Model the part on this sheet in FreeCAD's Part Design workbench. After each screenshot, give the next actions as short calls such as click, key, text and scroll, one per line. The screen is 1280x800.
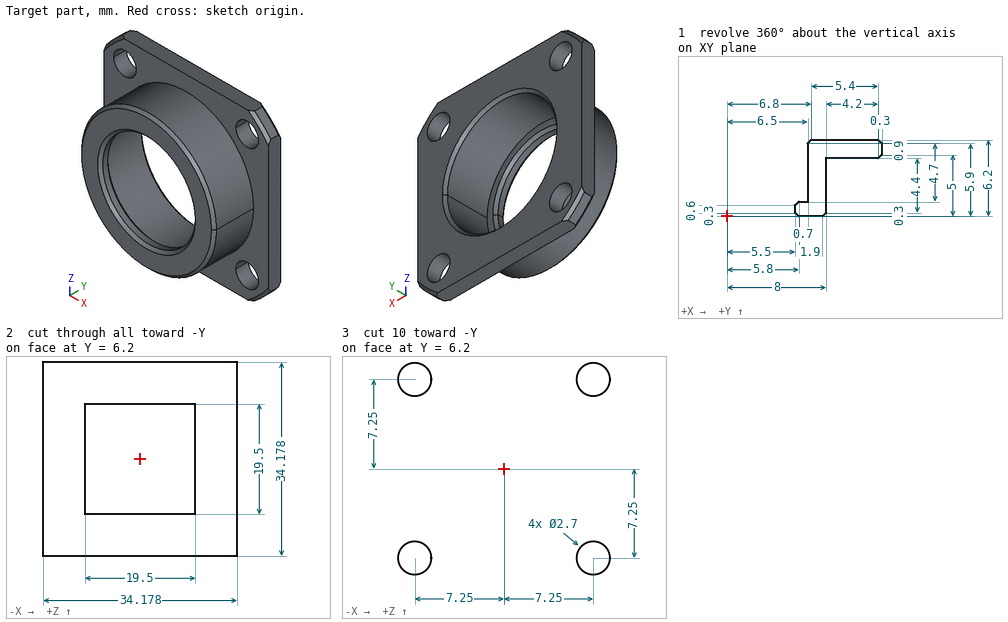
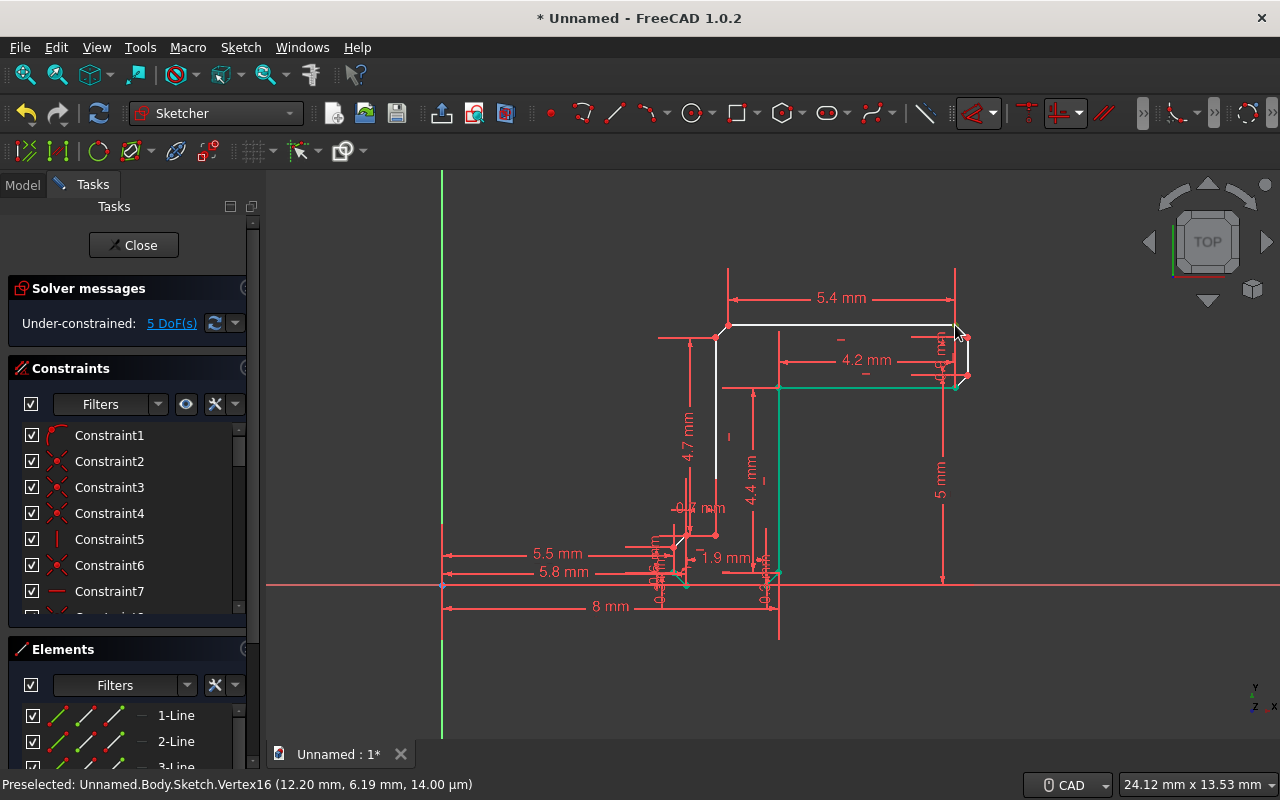
click(996, 114)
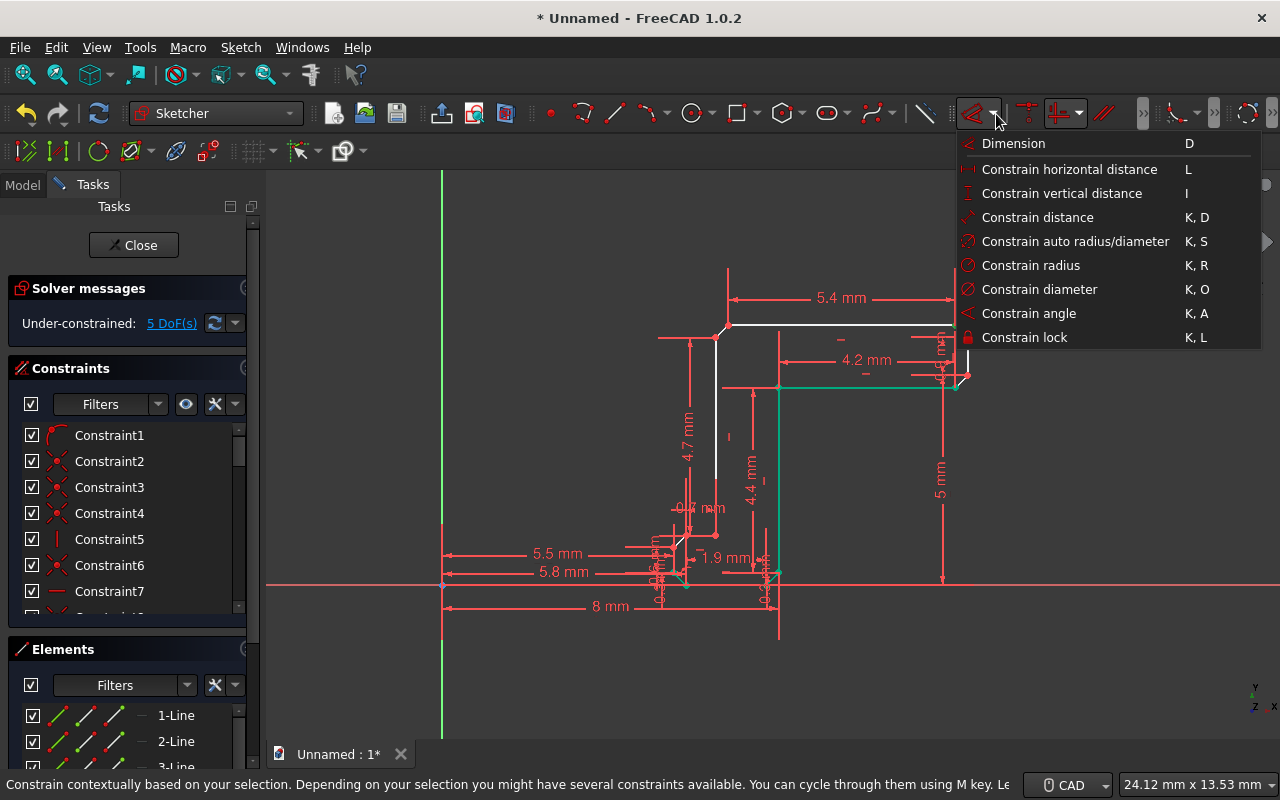
click(1109, 193)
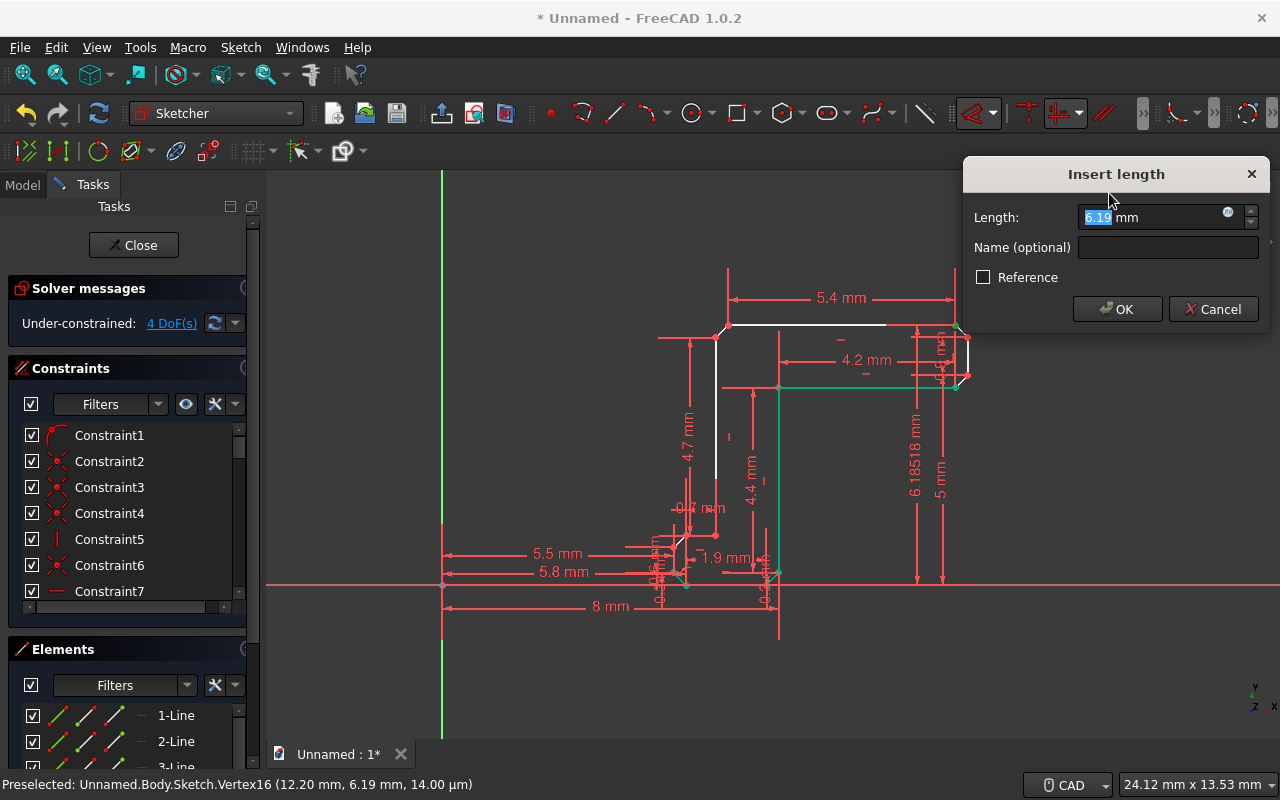
text(6.2)
key(Return)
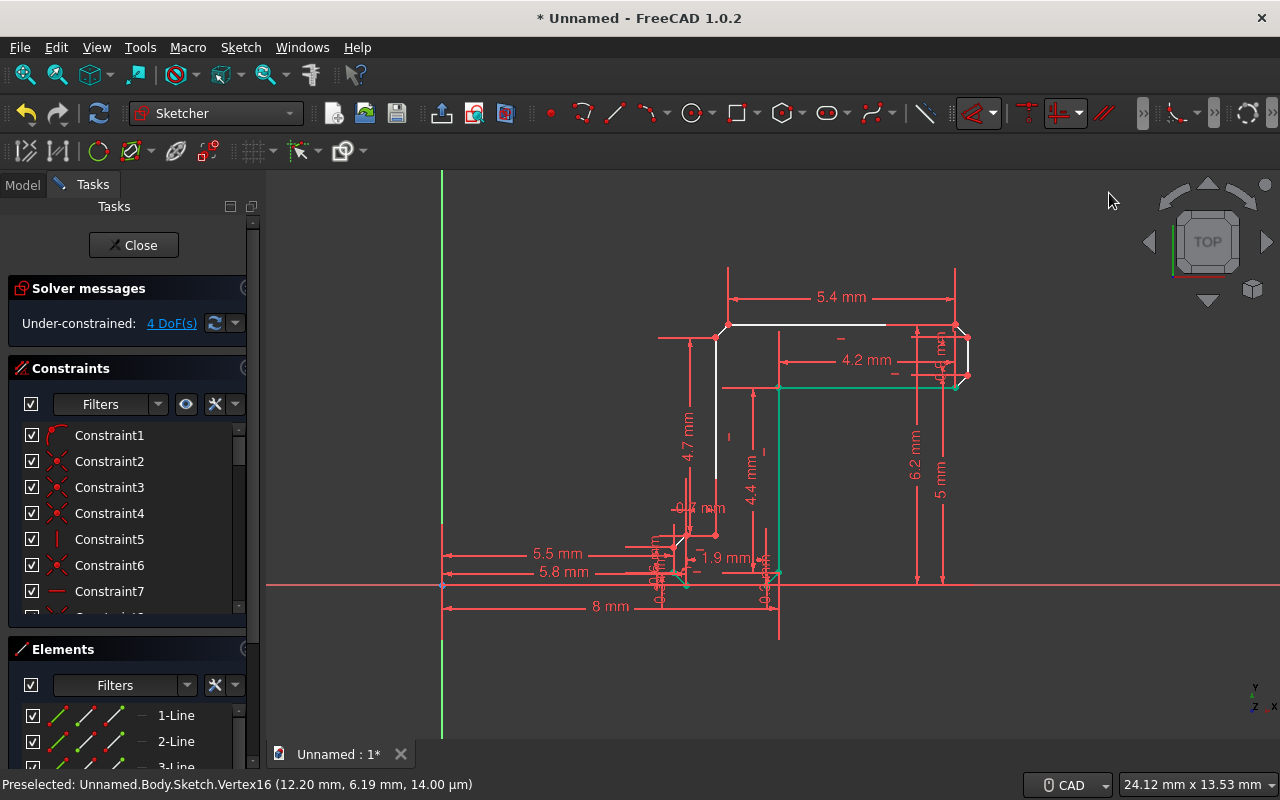
click(728, 325)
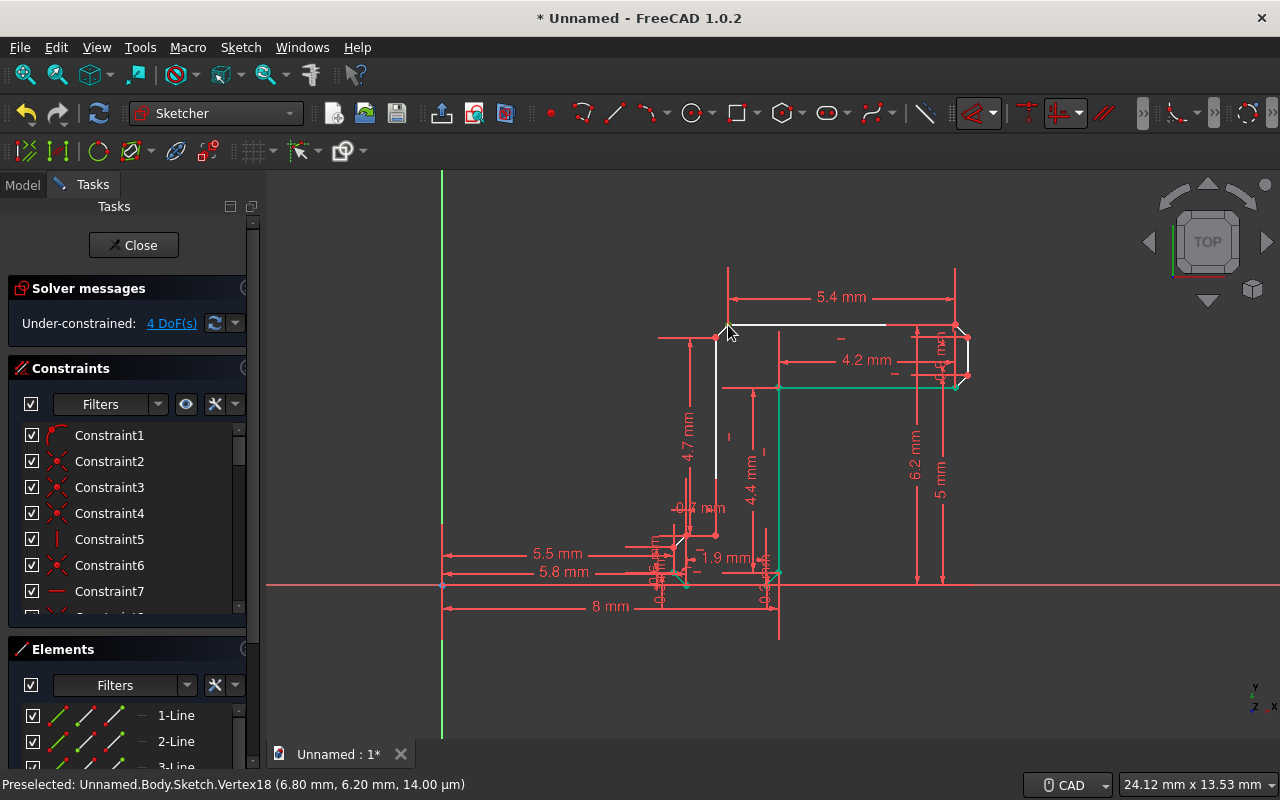
key(l)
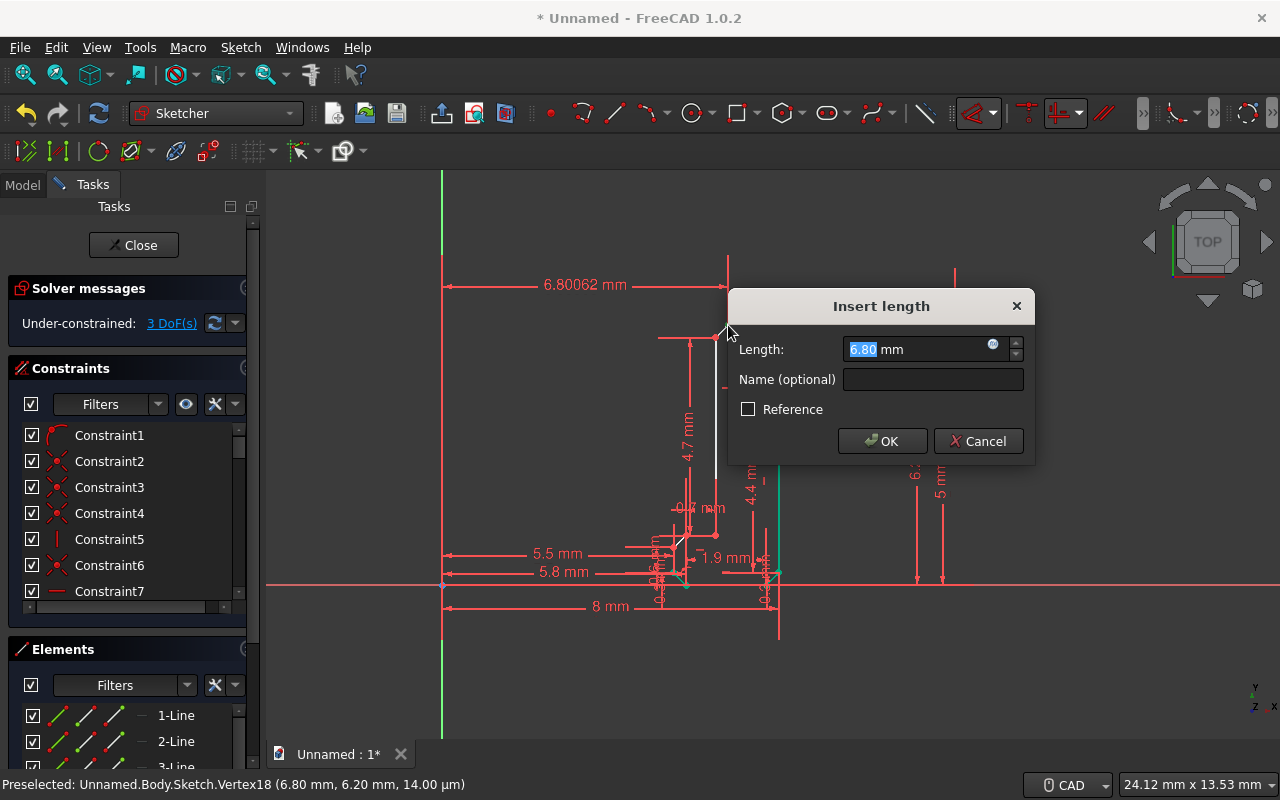
text(6.8)
key(Return)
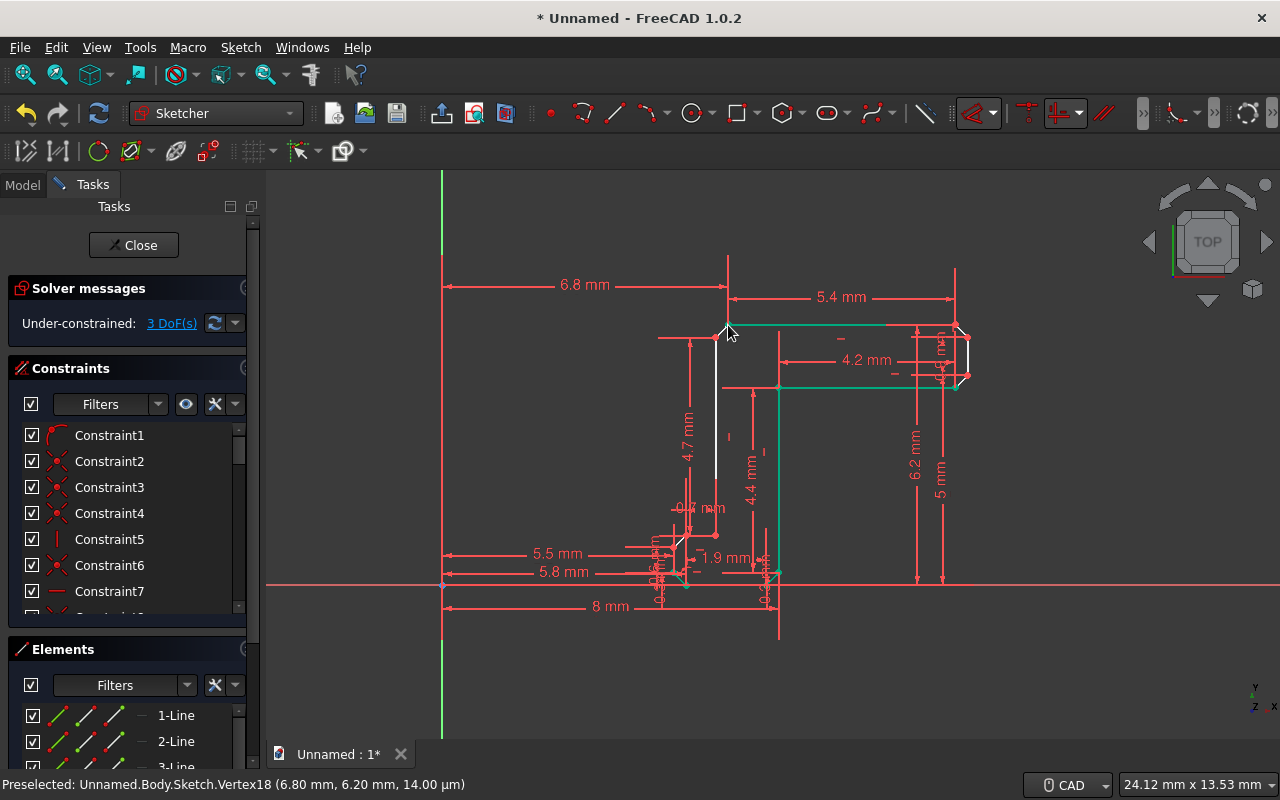
click(716, 338)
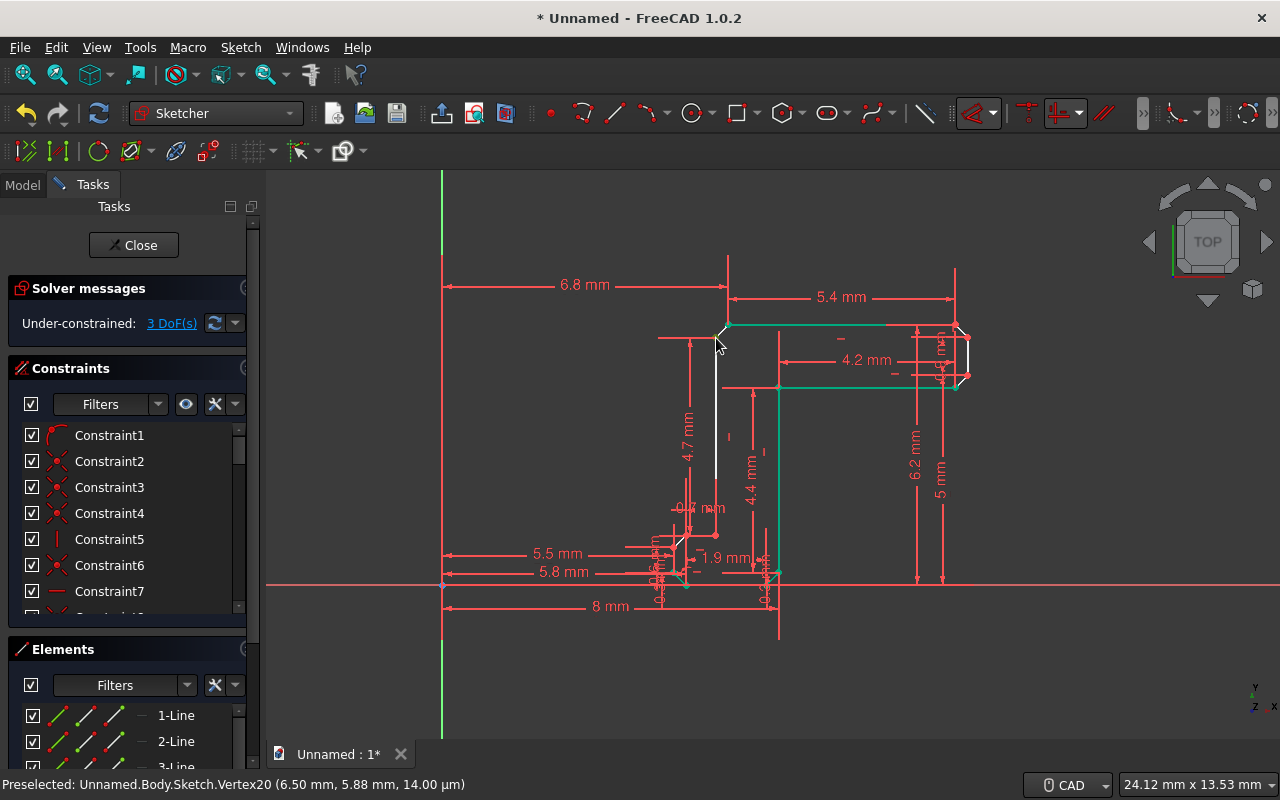
click(996, 114)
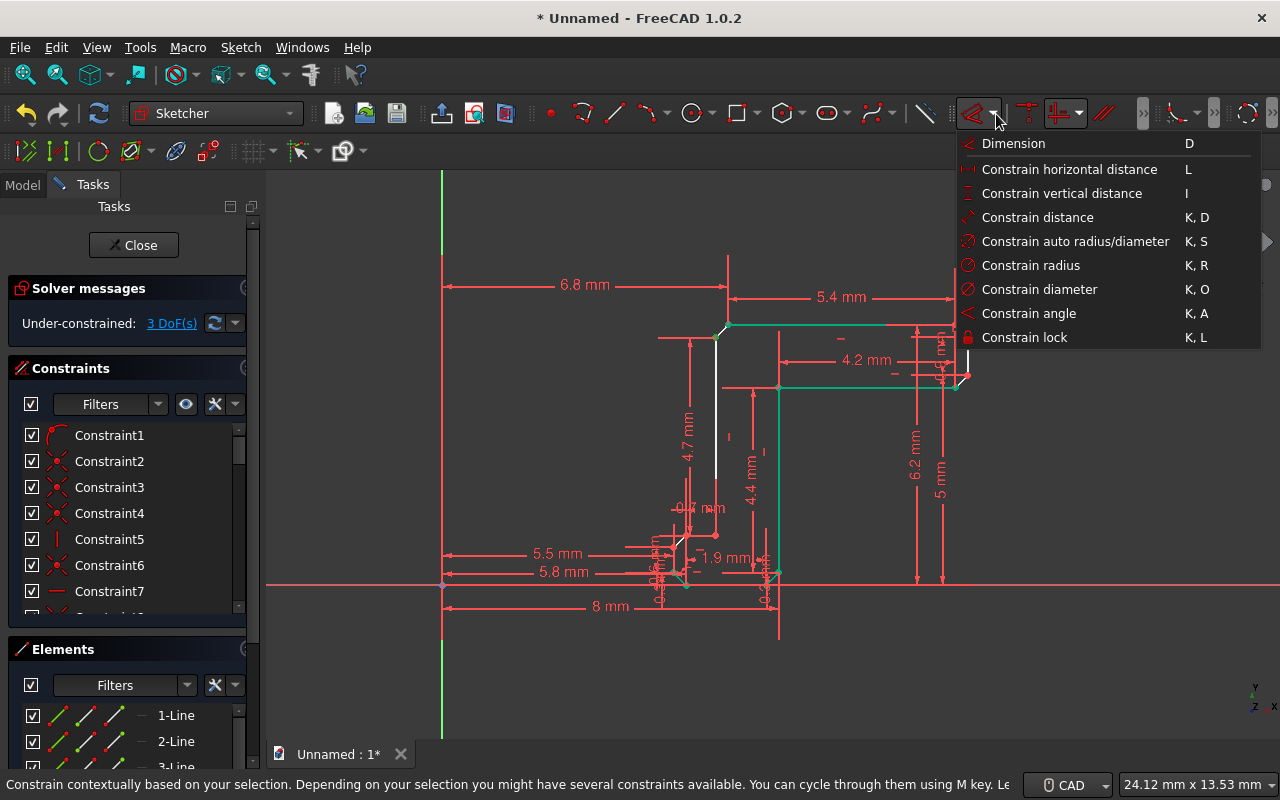
click(1109, 169)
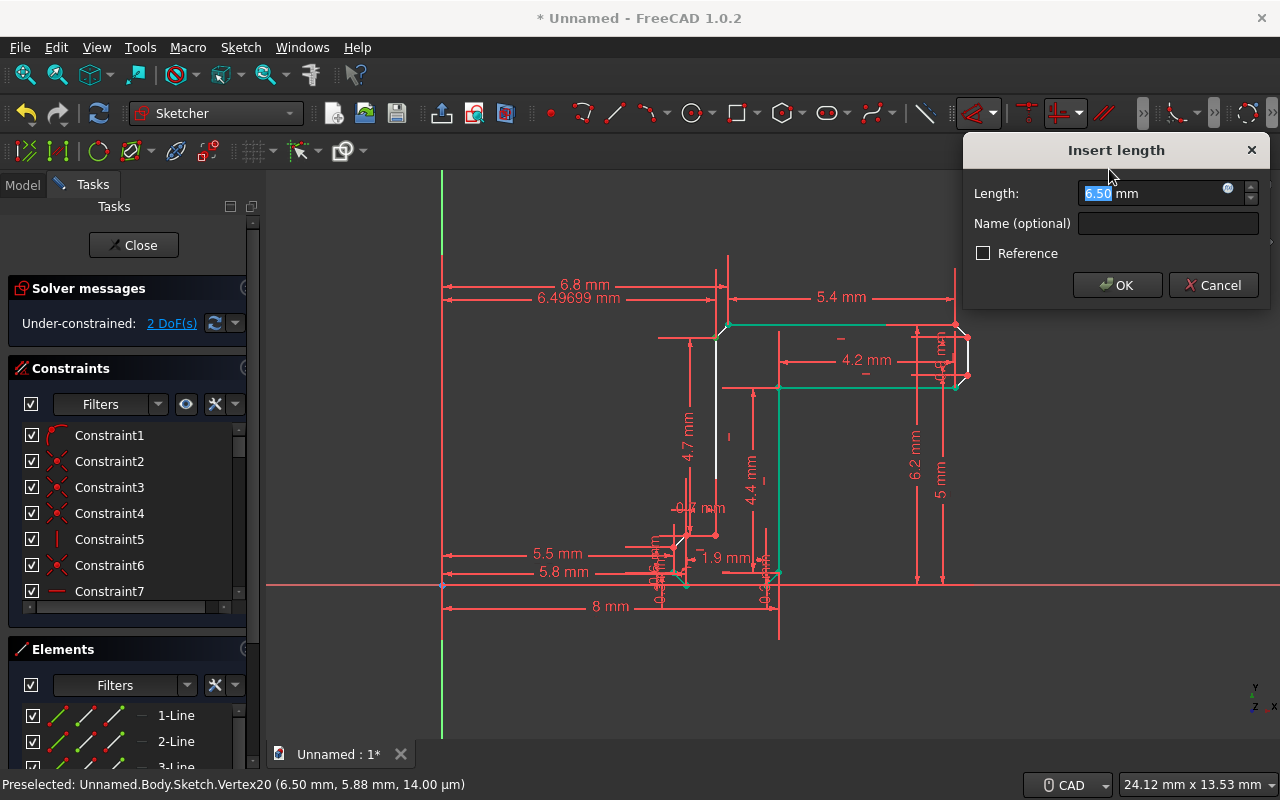
text(6.5)
key(Return)